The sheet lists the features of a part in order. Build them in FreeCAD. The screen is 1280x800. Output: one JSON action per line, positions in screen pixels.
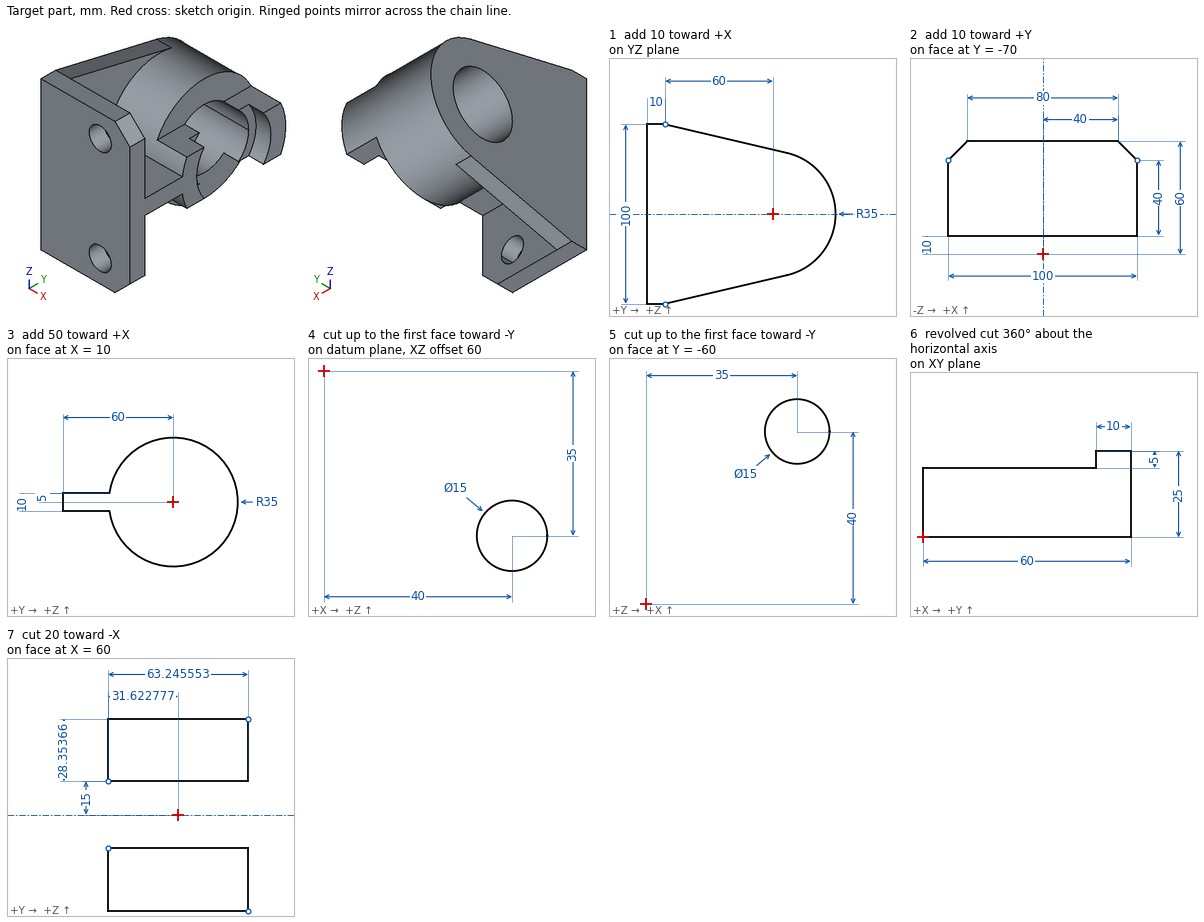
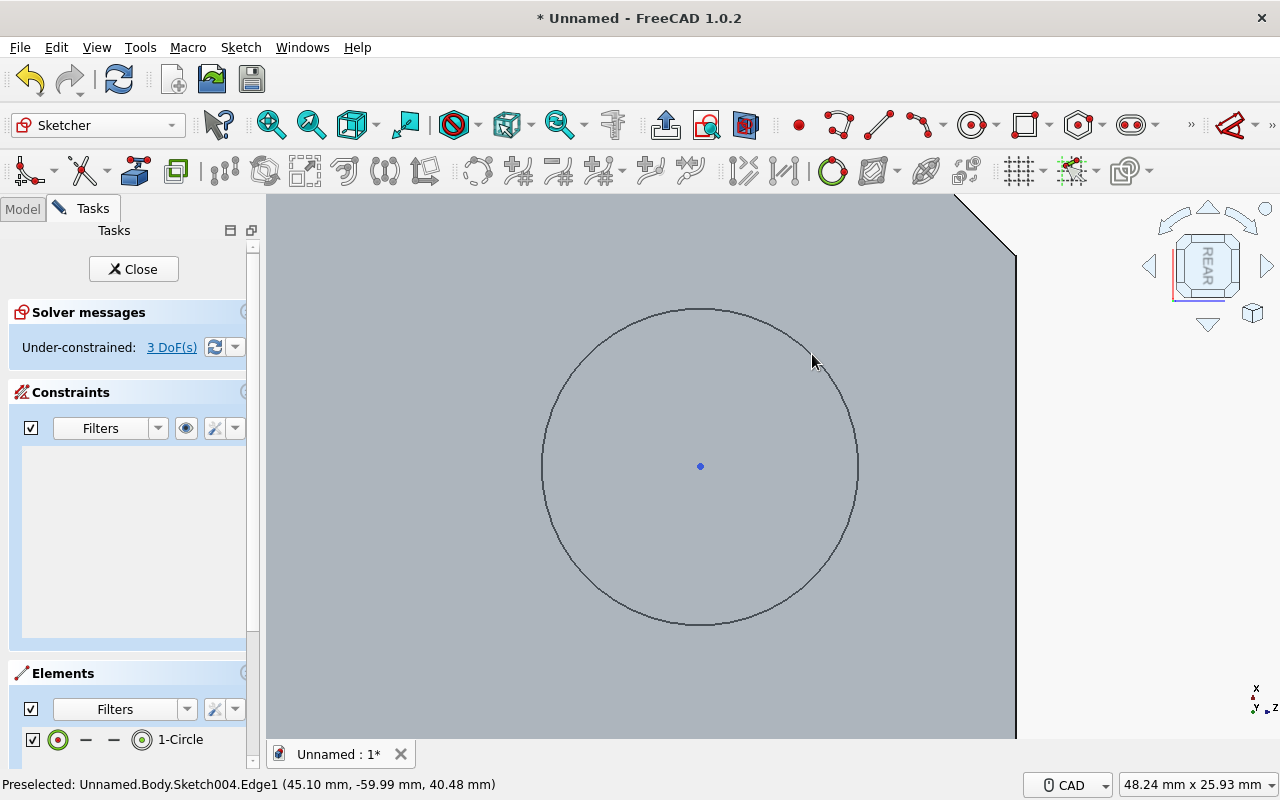
{"action": "left_click", "coordinate": [1230, 126]}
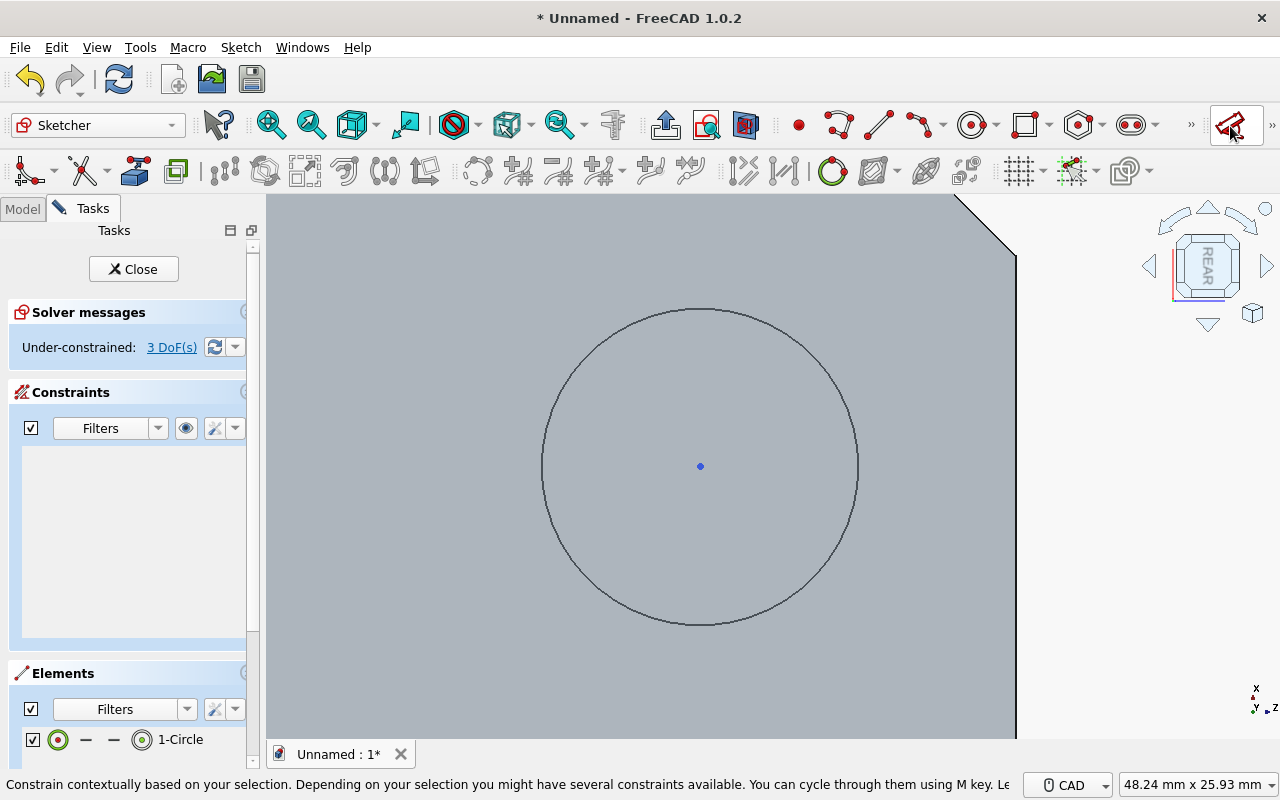
{"action": "left_click", "coordinate": [812, 355]}
{"action": "left_click", "coordinate": [835, 332]}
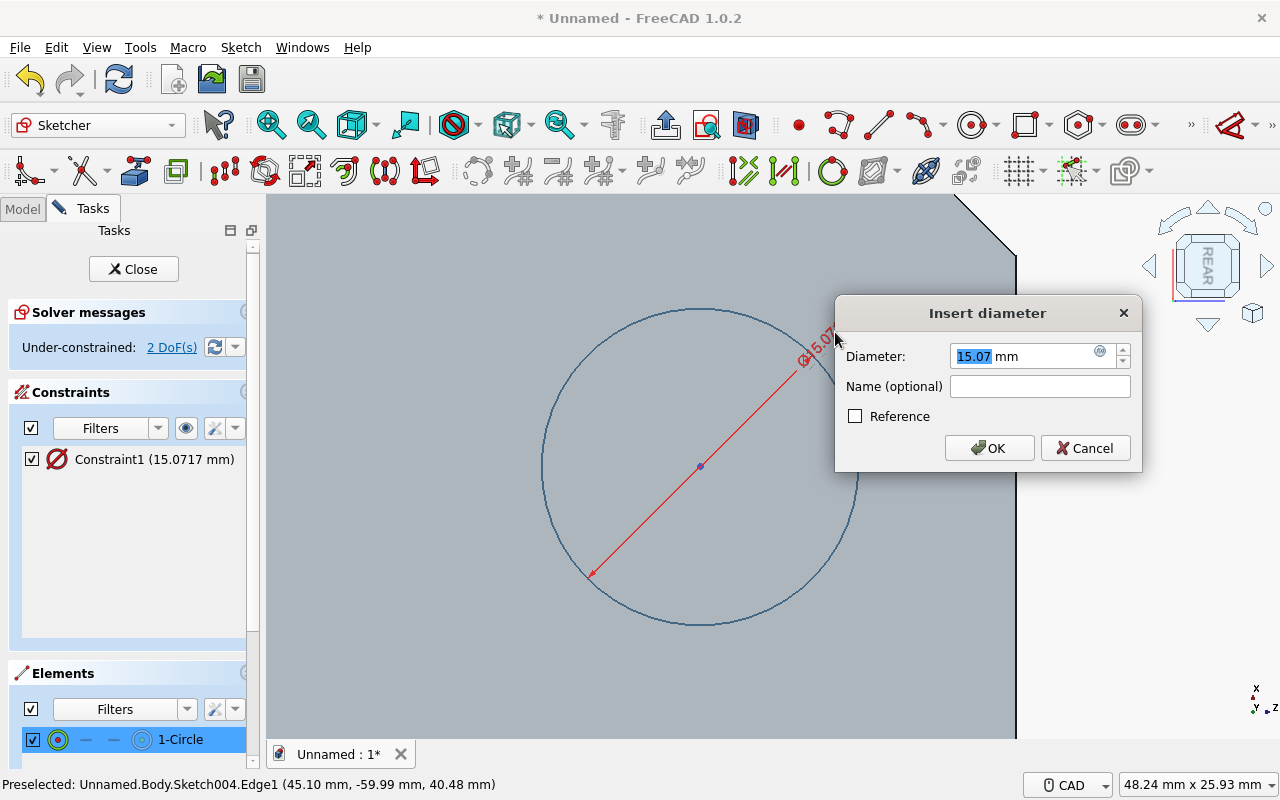
{"action": "type", "text": "15"}
{"action": "key", "text": "Return"}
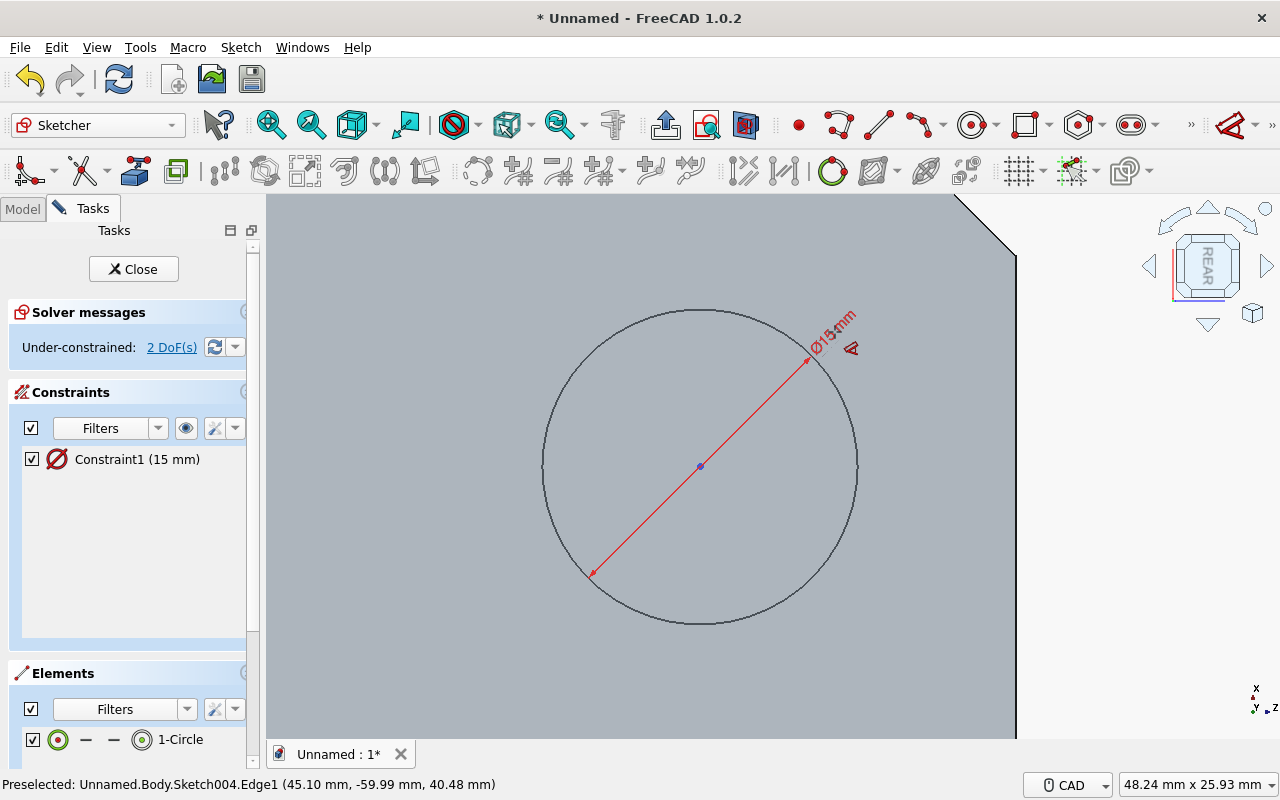
{"action": "left_click", "coordinate": [700, 467]}
{"action": "left_click", "coordinate": [497, 433]}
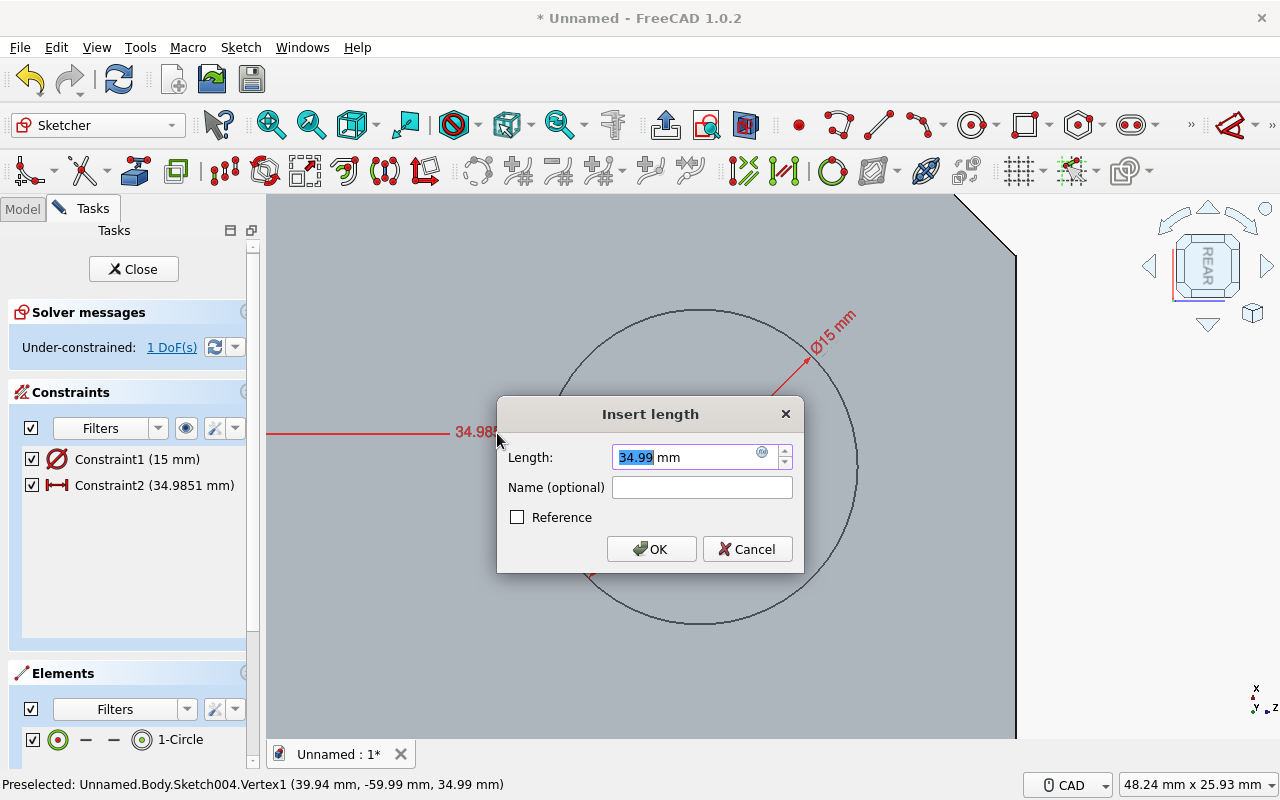
{"action": "type", "text": "35"}
{"action": "key", "text": "Return"}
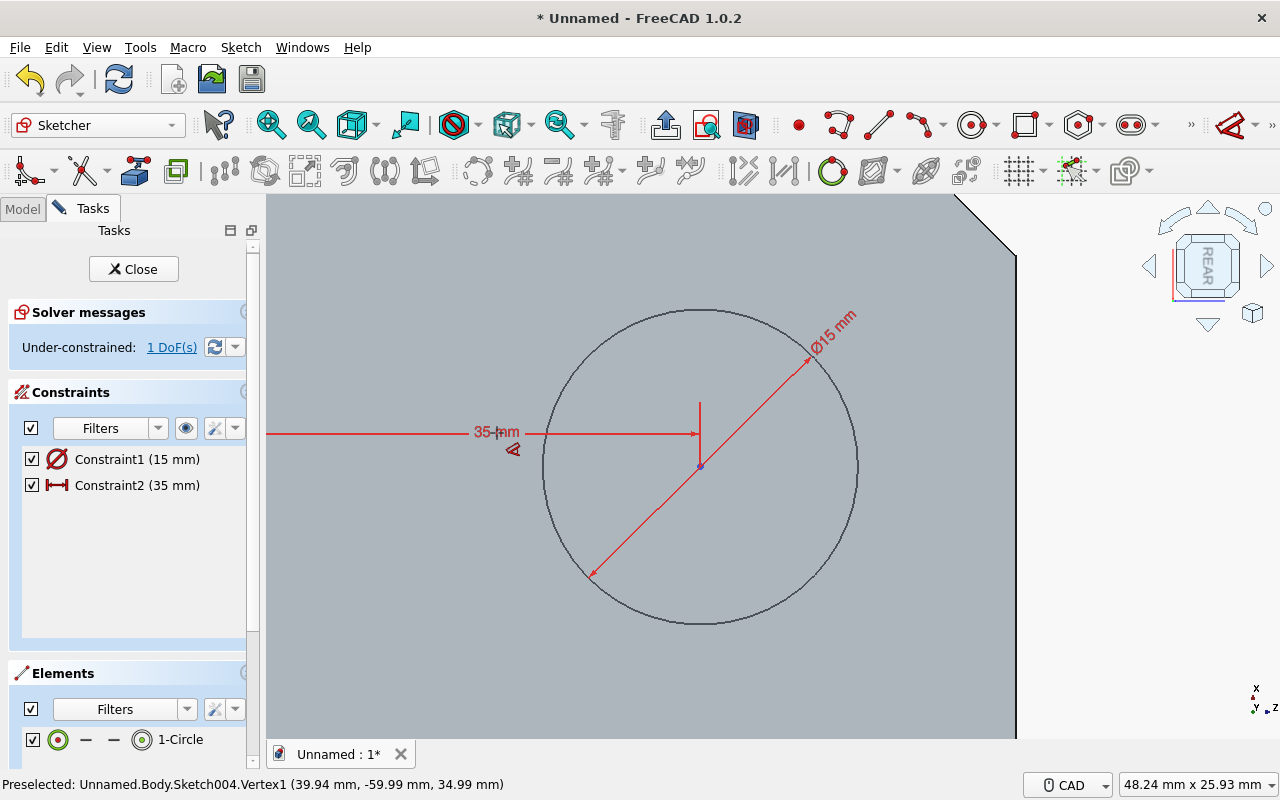
{"action": "left_click", "coordinate": [700, 467]}
{"action": "left_click", "coordinate": [734, 589]}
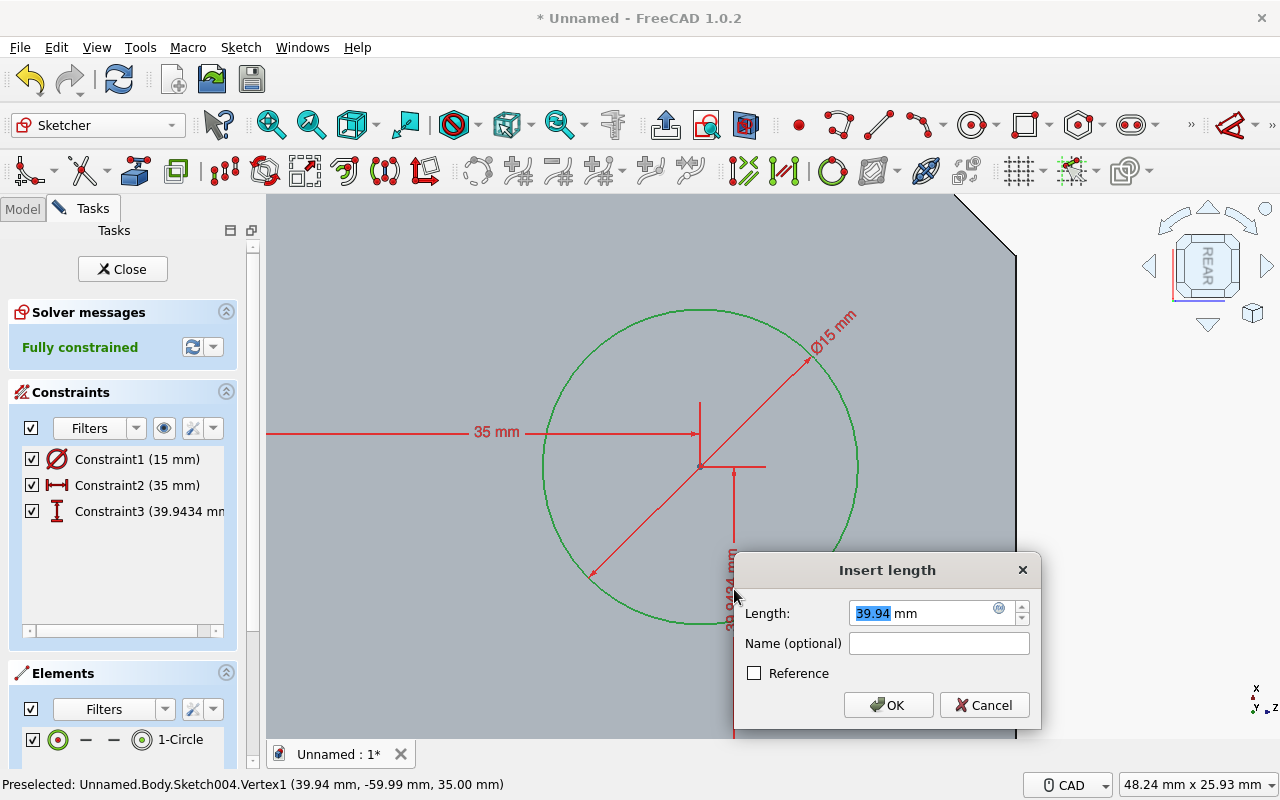
{"action": "type", "text": "40"}
{"action": "key", "text": "Return"}
{"action": "key", "text": "Escape"}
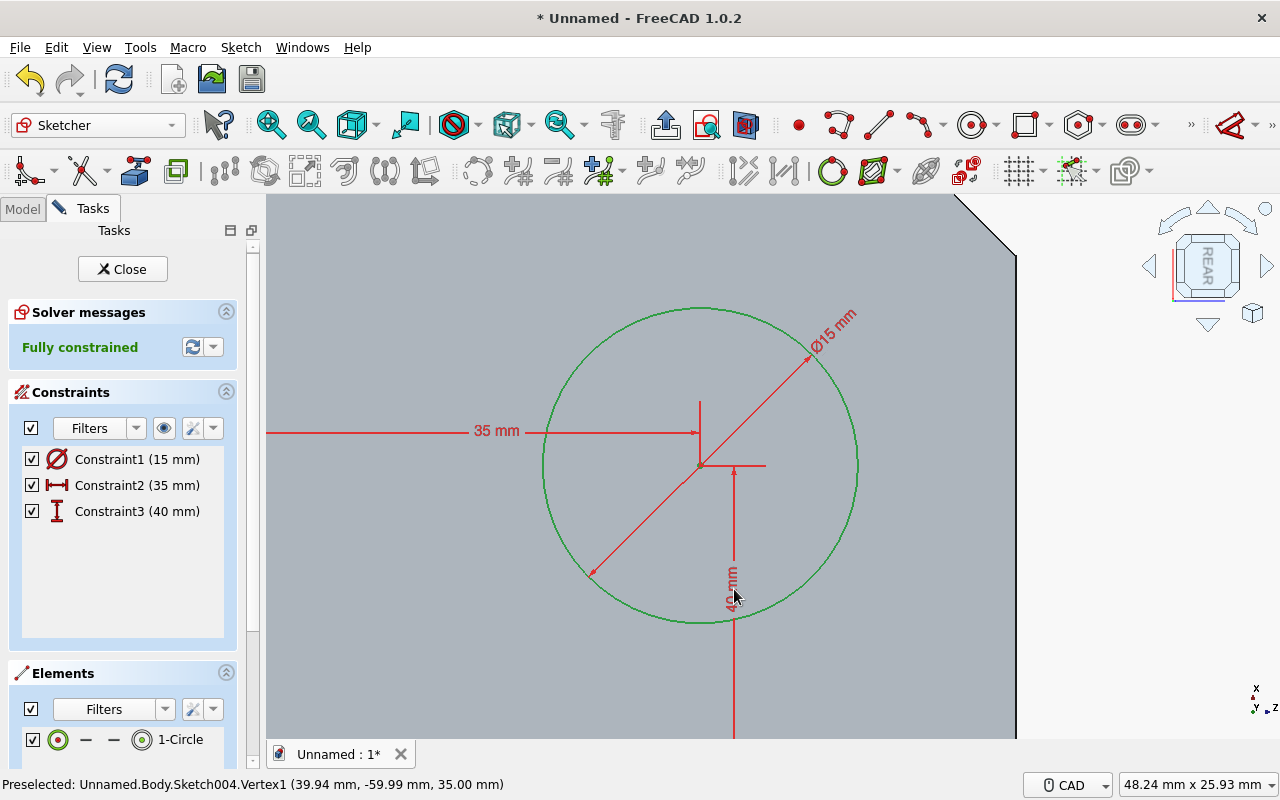
{"action": "left_click", "coordinate": [123, 269]}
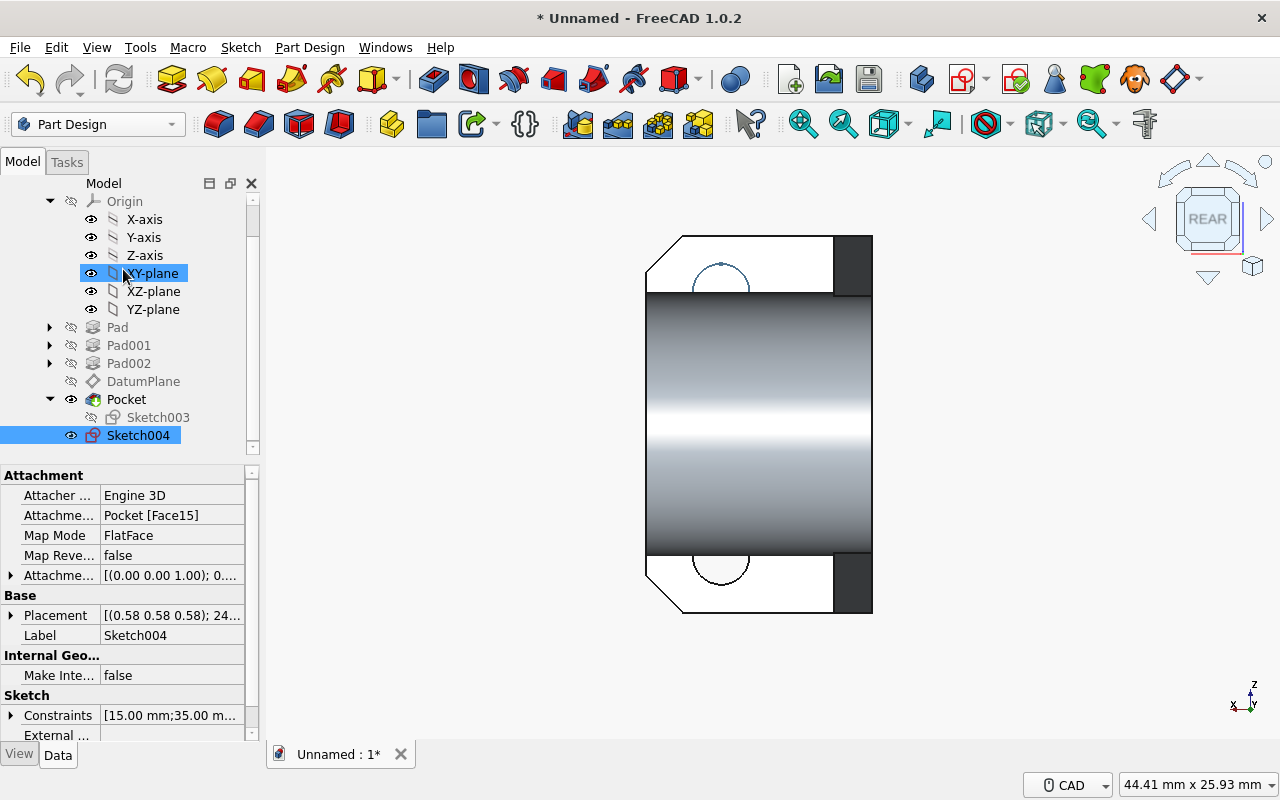
{"action": "left_click", "coordinate": [434, 80]}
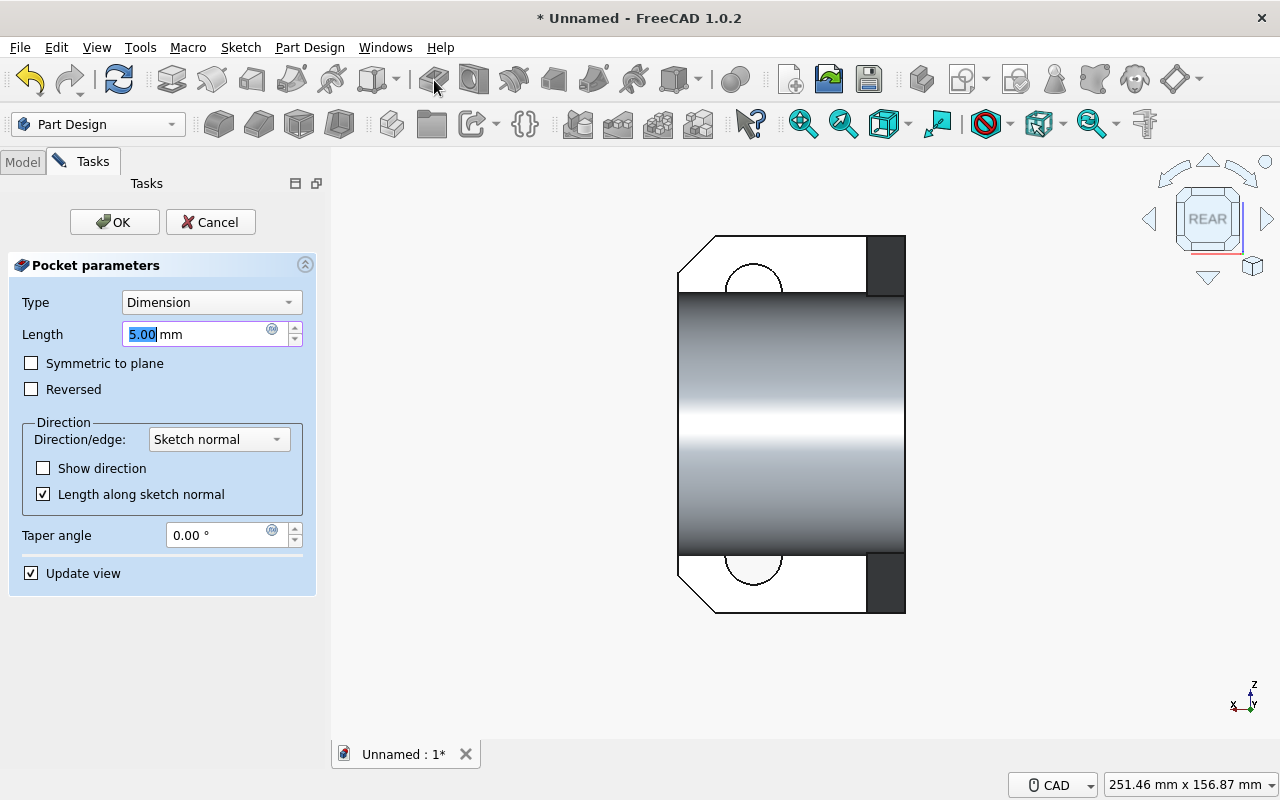
{"action": "left_click", "coordinate": [212, 302]}